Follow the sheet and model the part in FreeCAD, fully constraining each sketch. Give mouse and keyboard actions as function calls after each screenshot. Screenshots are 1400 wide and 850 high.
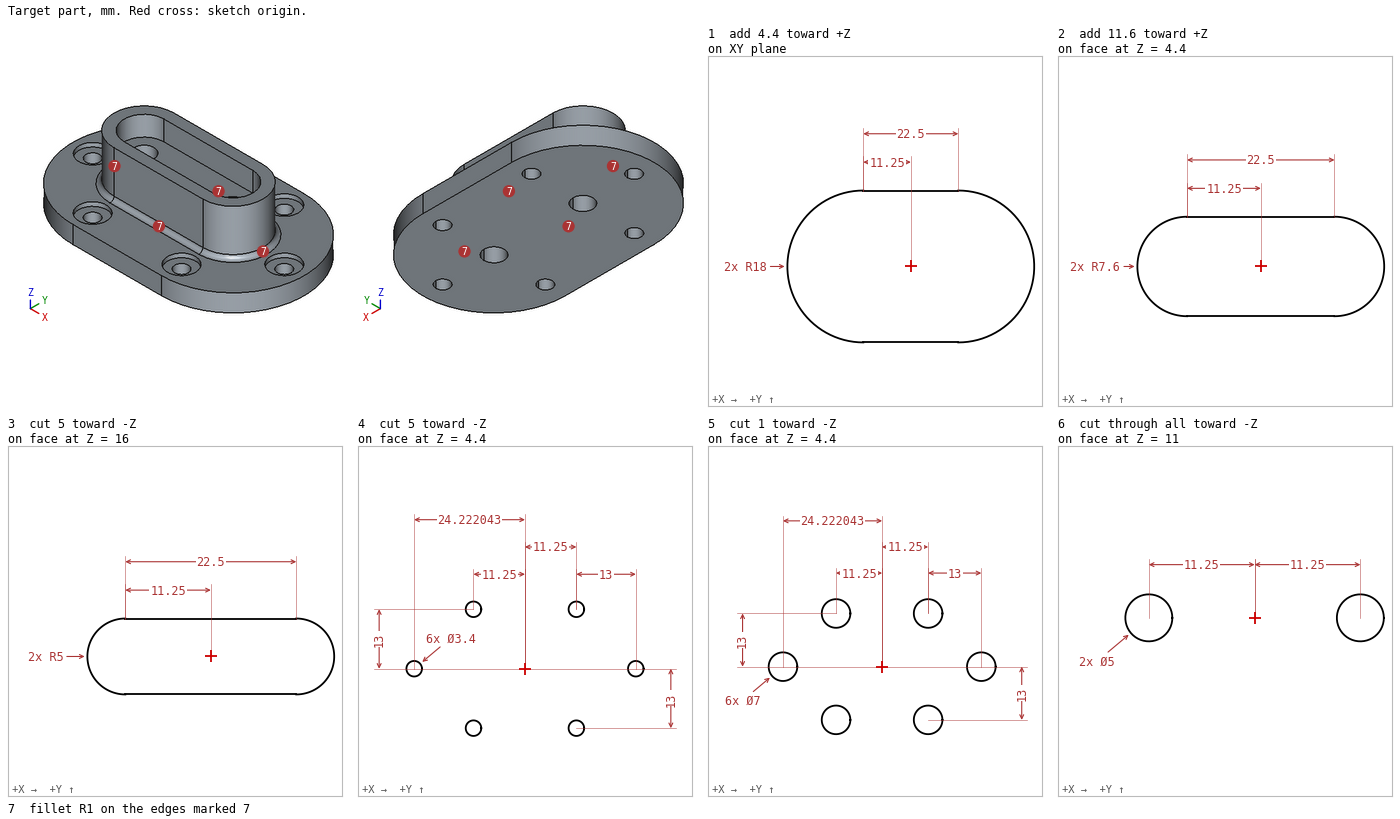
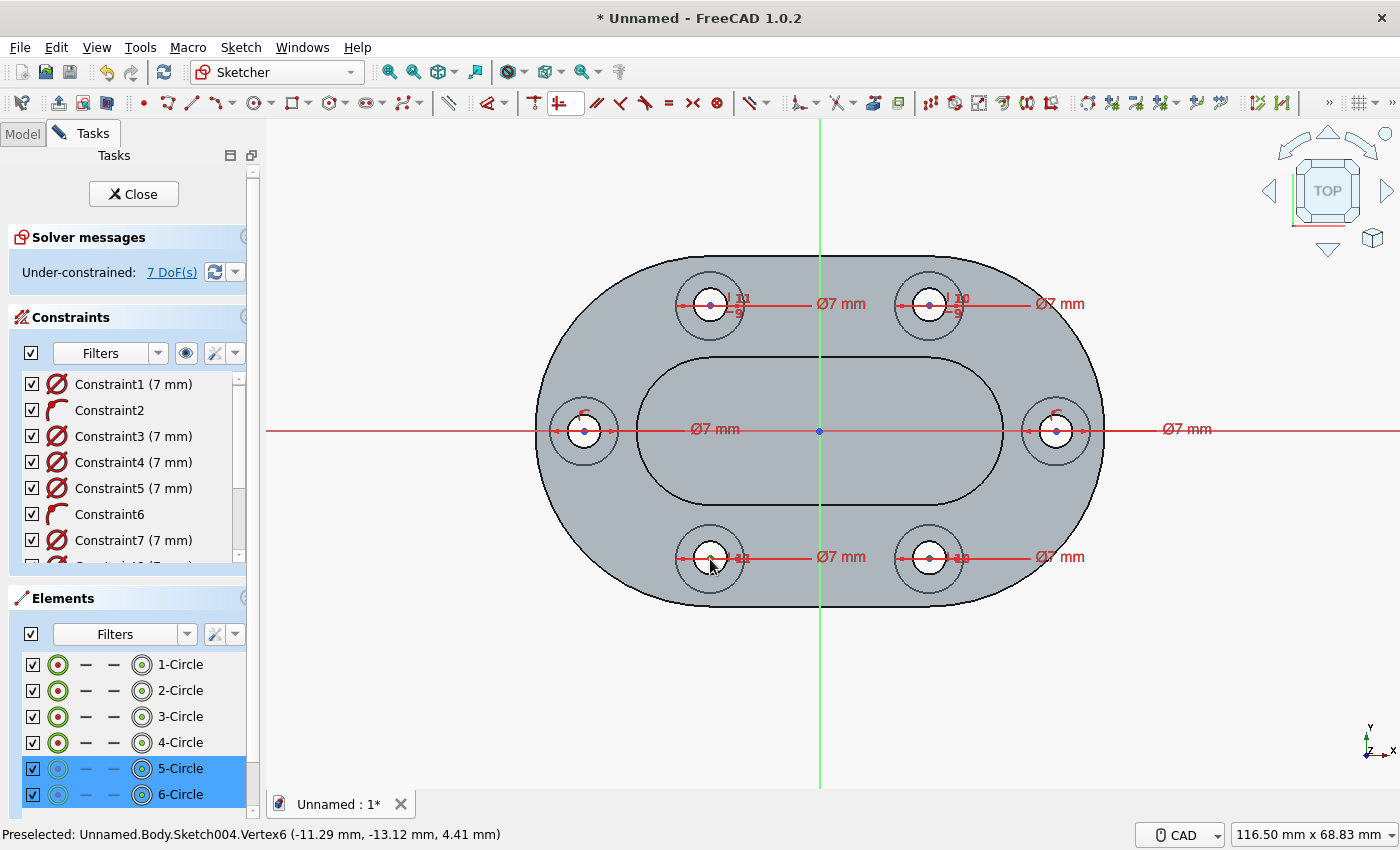
key(h)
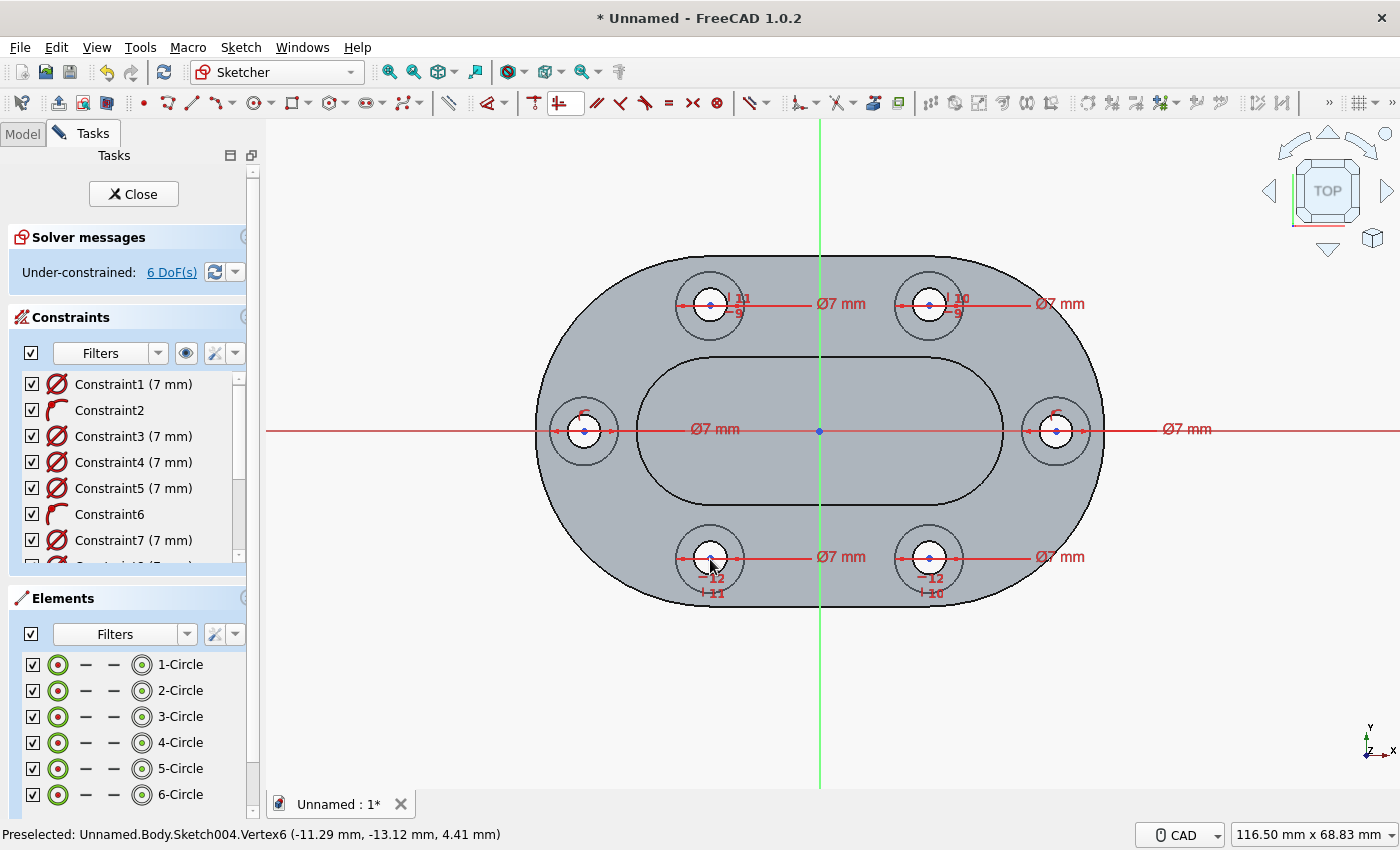
click(488, 104)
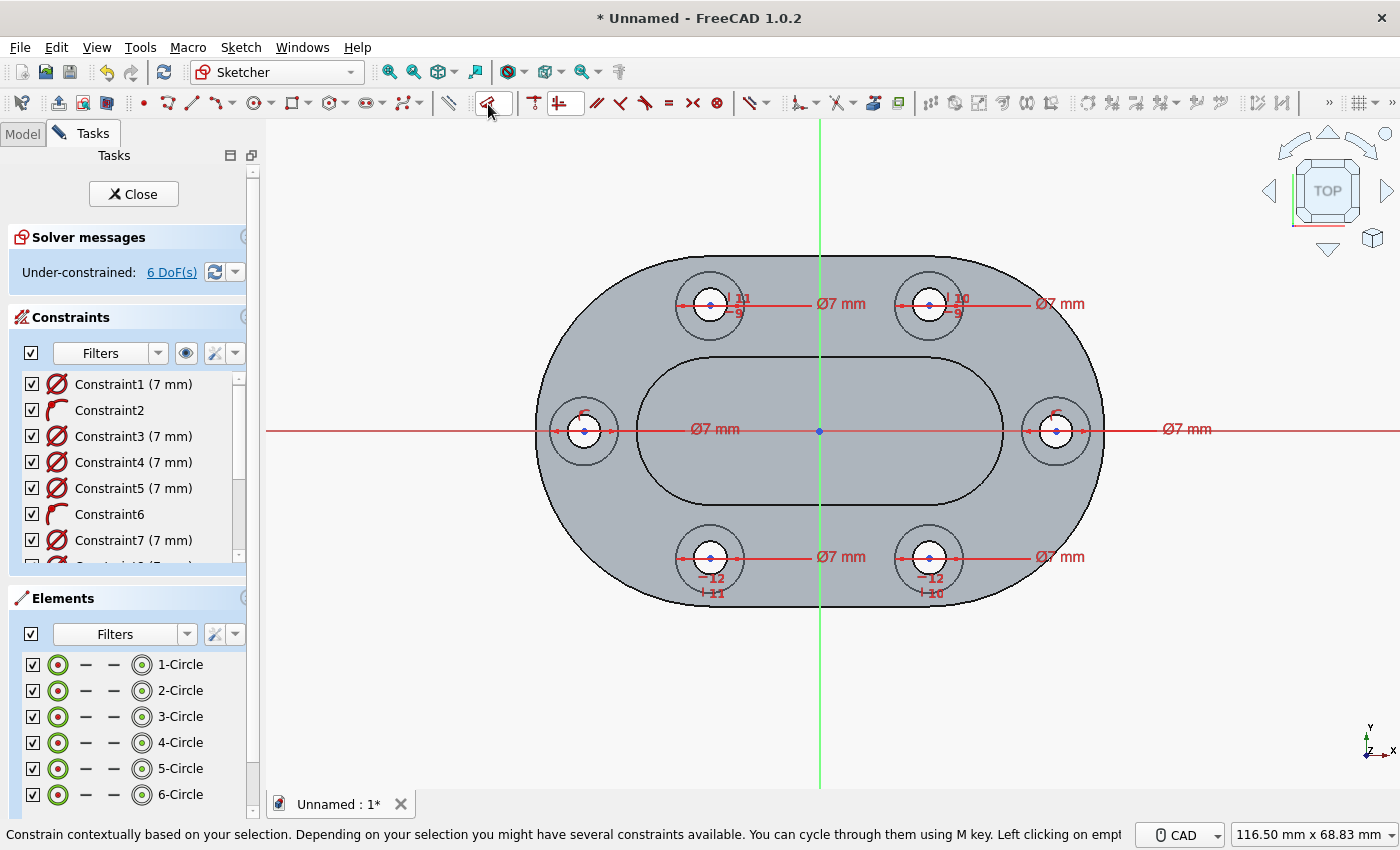
click(710, 306)
click(676, 369)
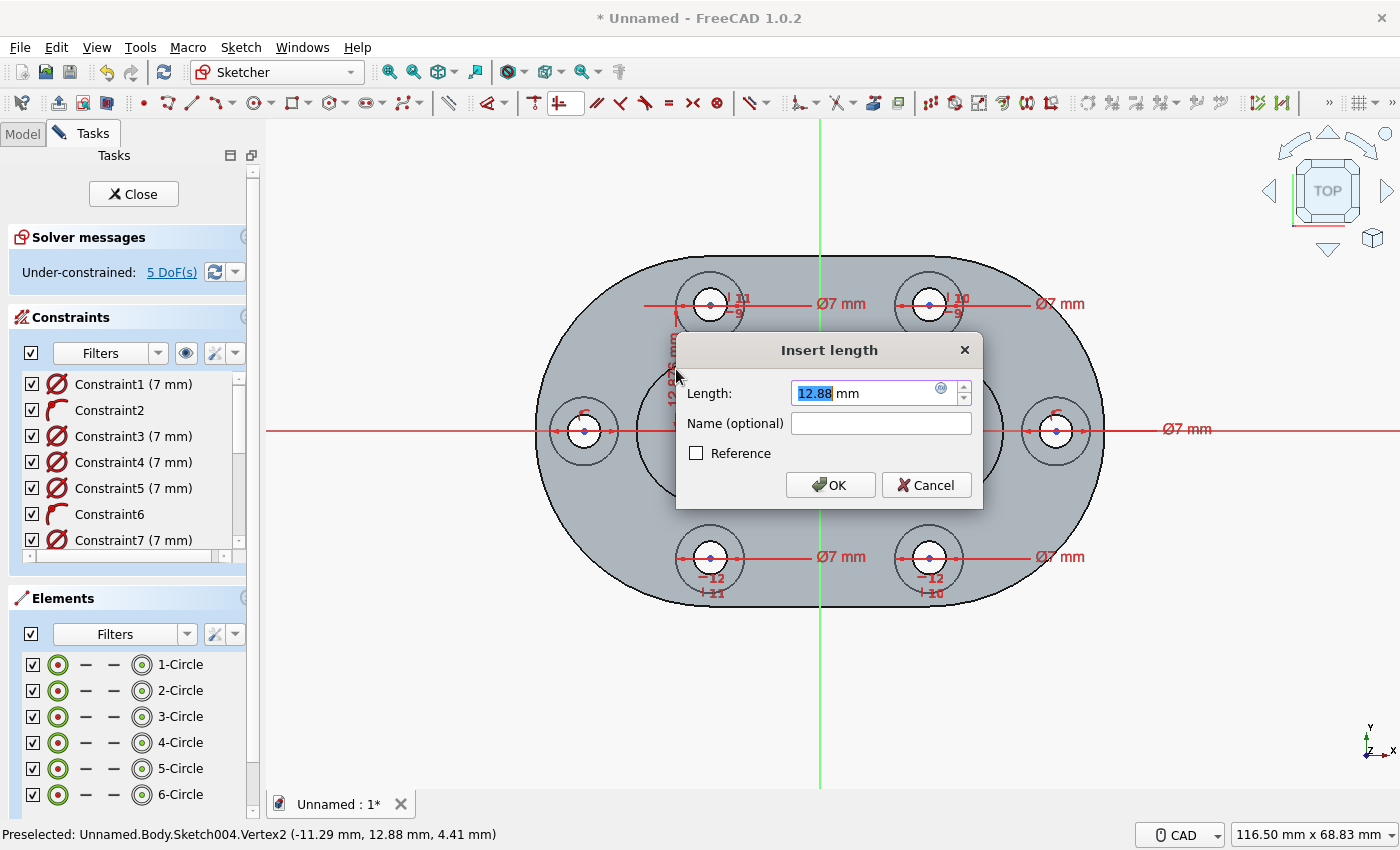
text(13)
key(Return)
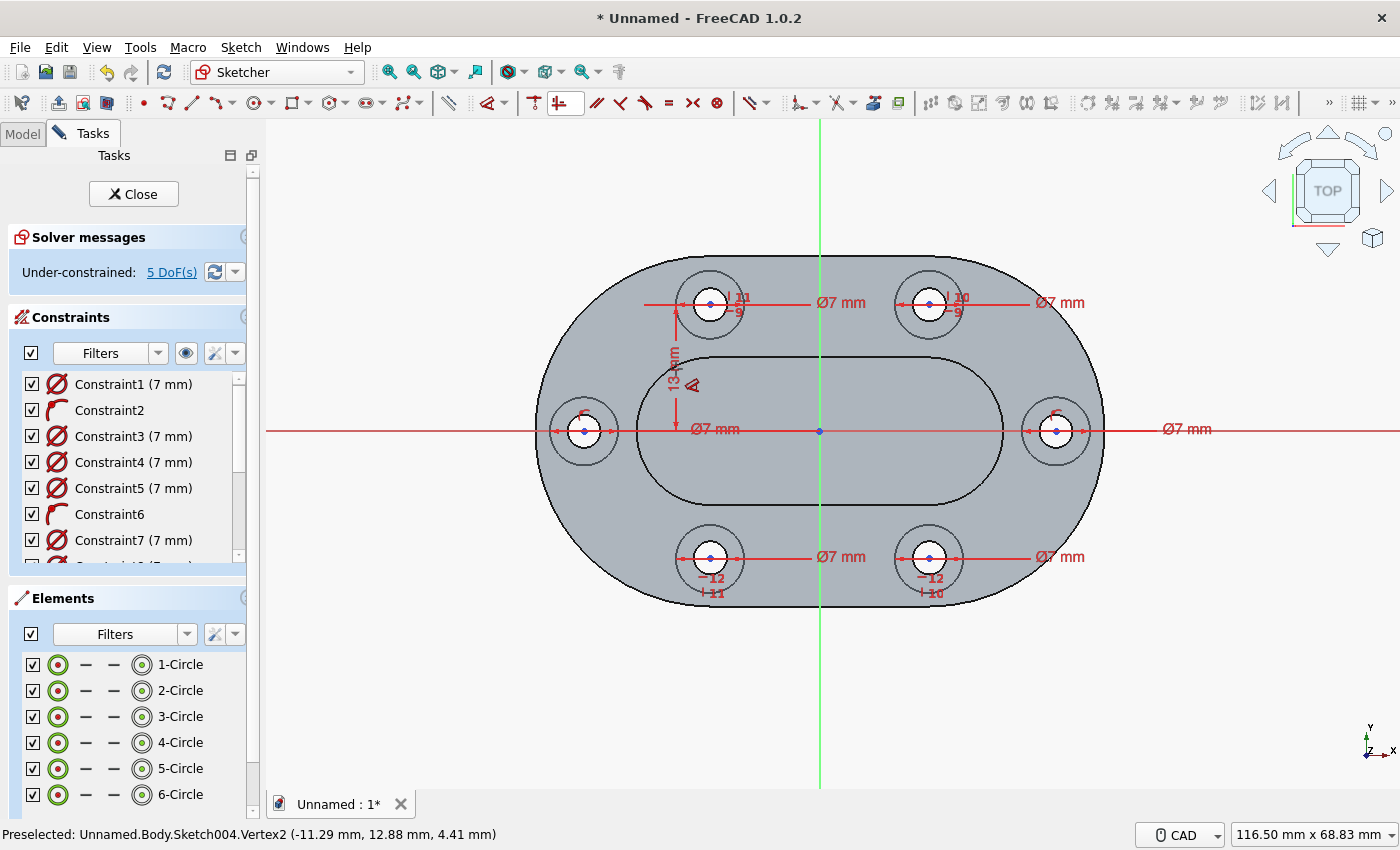
click(929, 559)
click(963, 495)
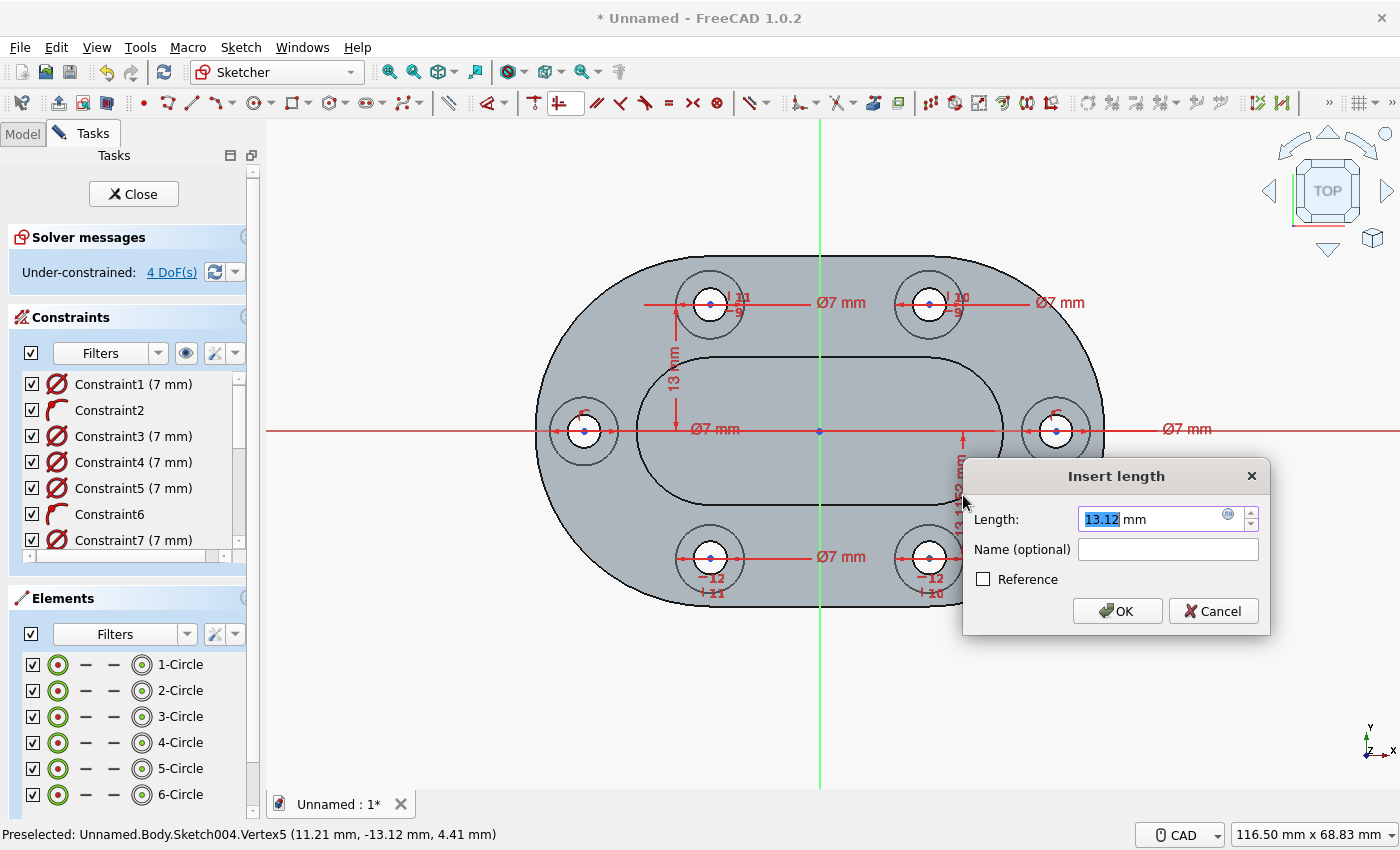
text(13)
key(Return)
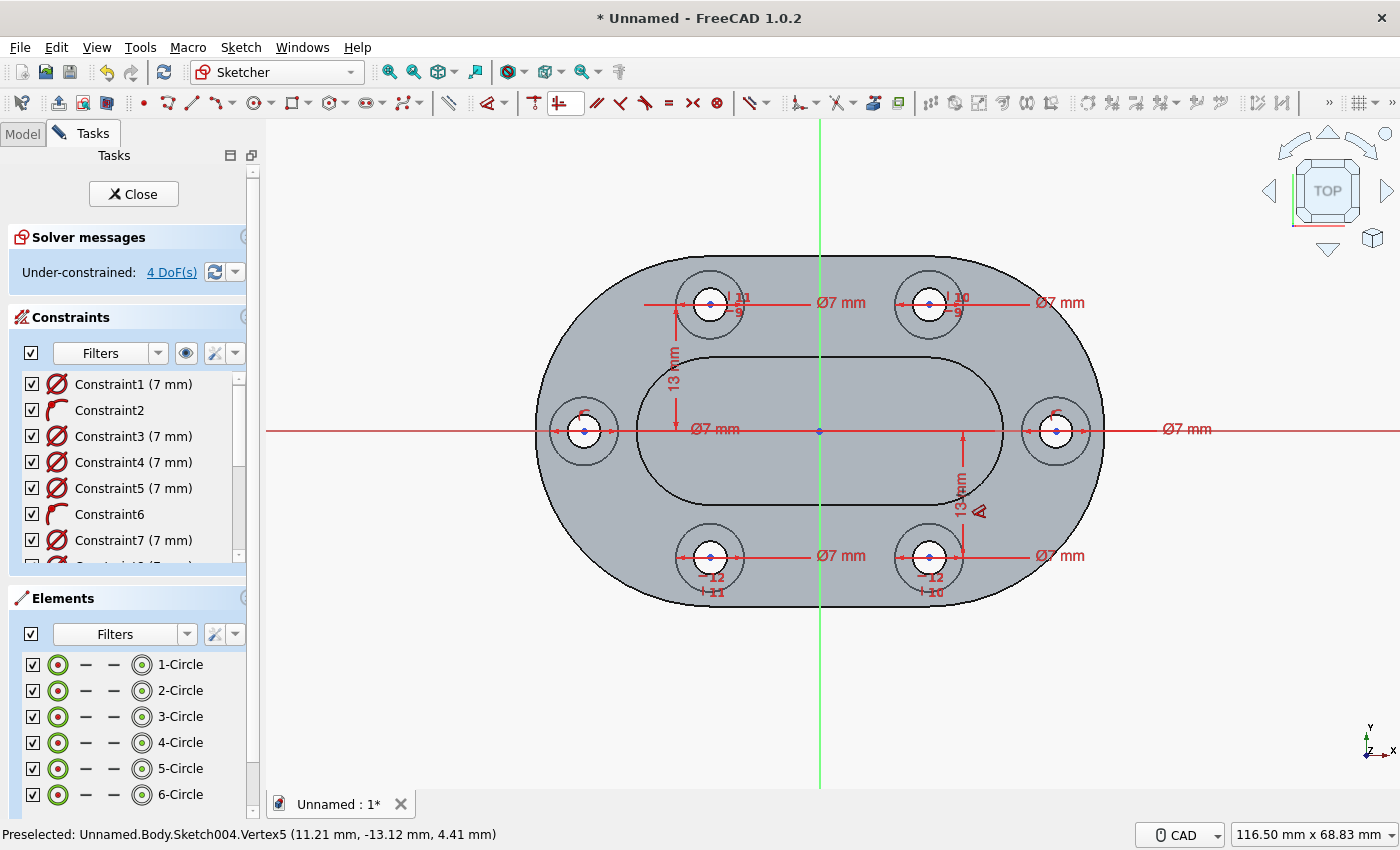
click(929, 305)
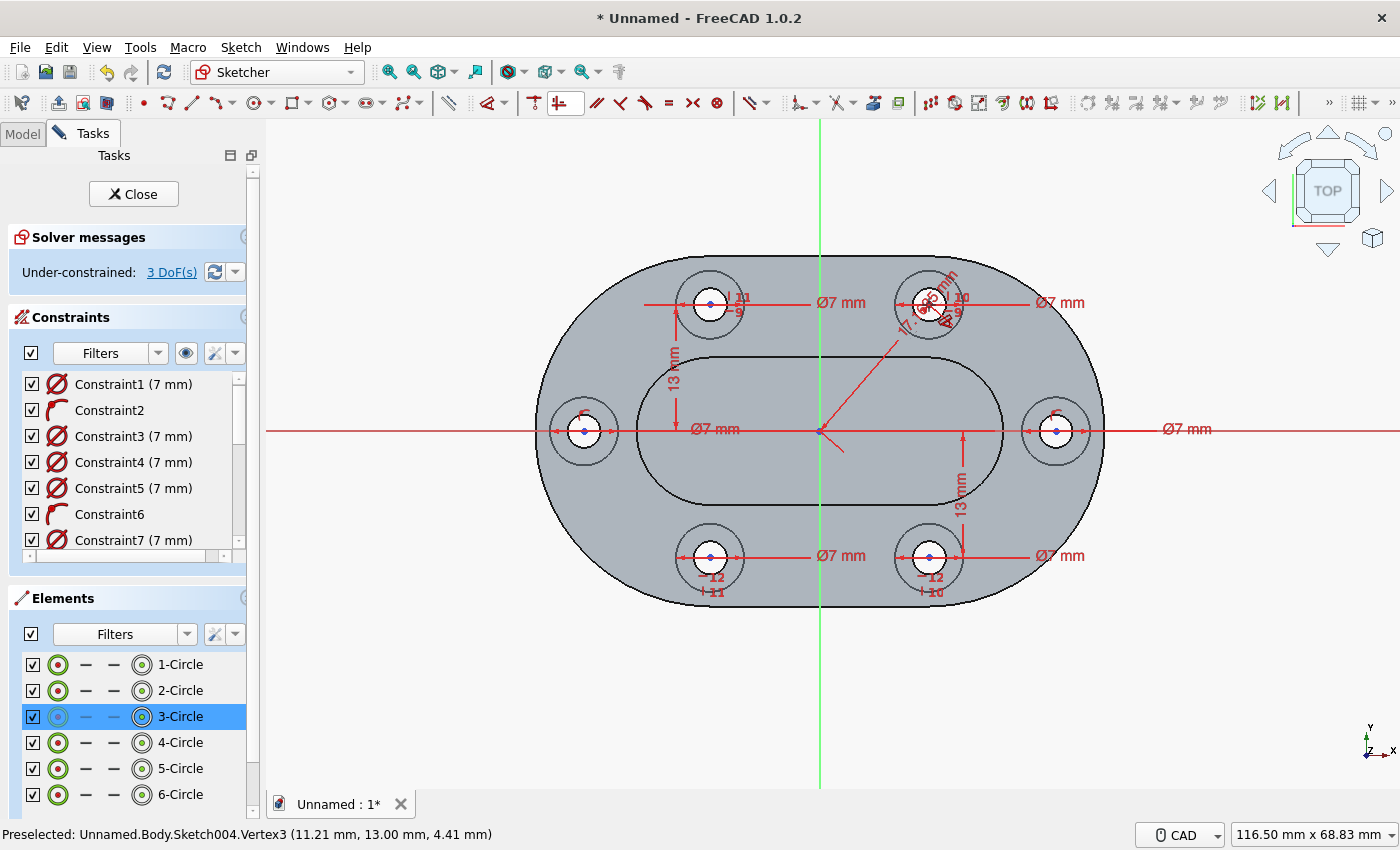
click(1056, 431)
click(992, 271)